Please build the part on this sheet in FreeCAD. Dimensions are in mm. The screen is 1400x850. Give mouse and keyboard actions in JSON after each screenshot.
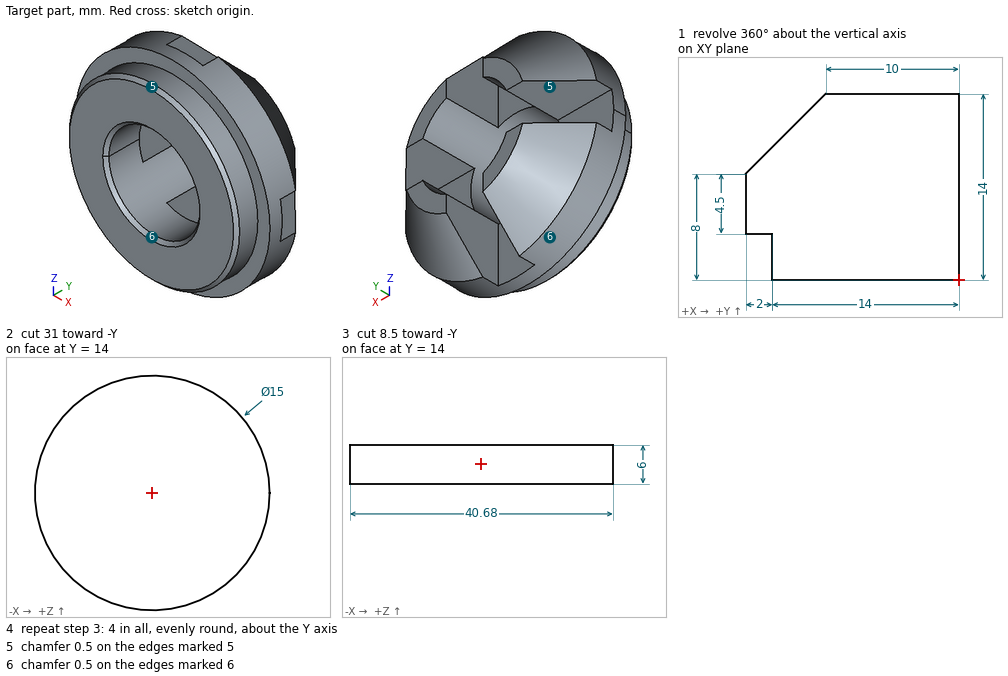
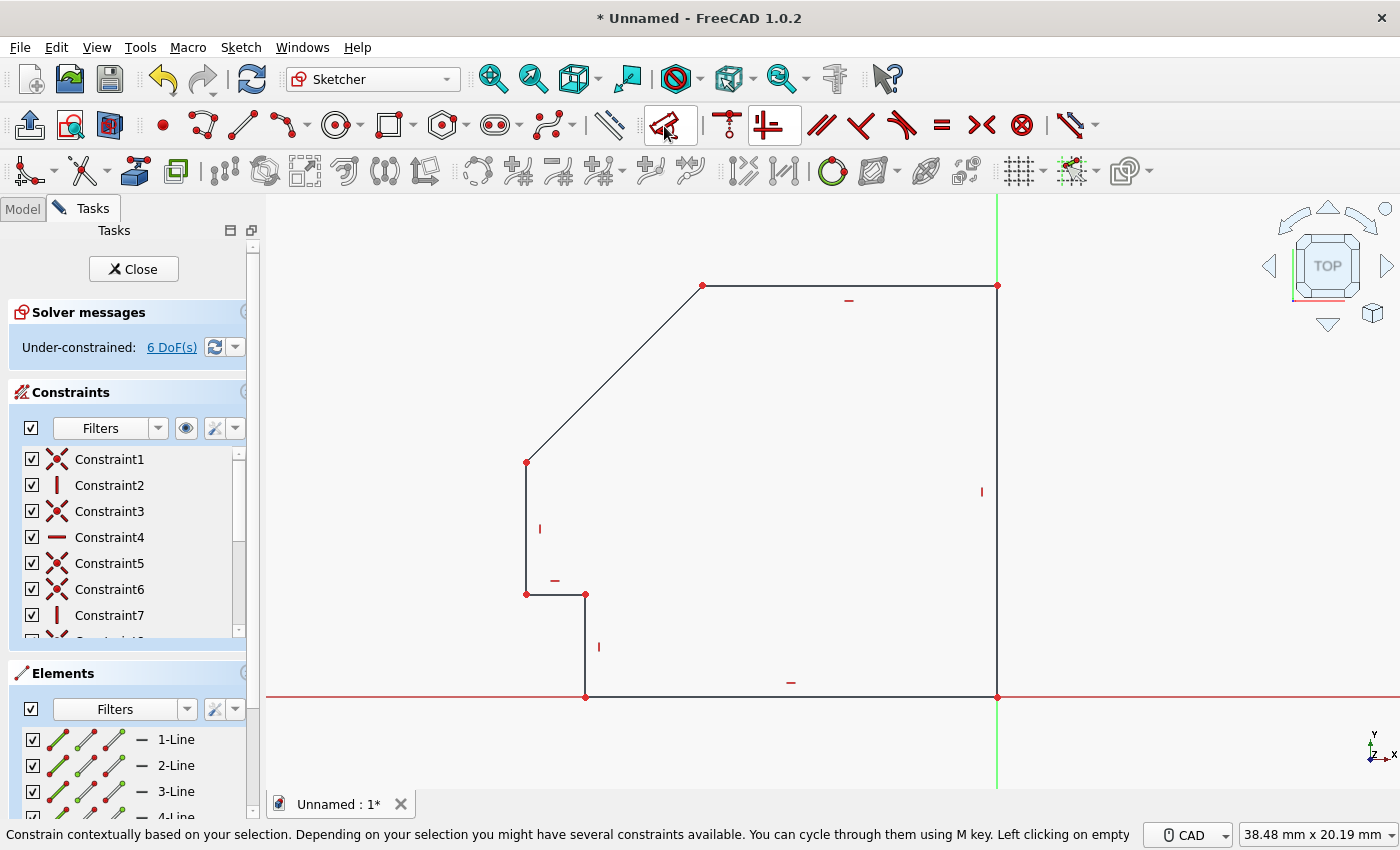
{"action": "left_click", "coordinate": [544, 595]}
{"action": "left_click", "coordinate": [555, 629]}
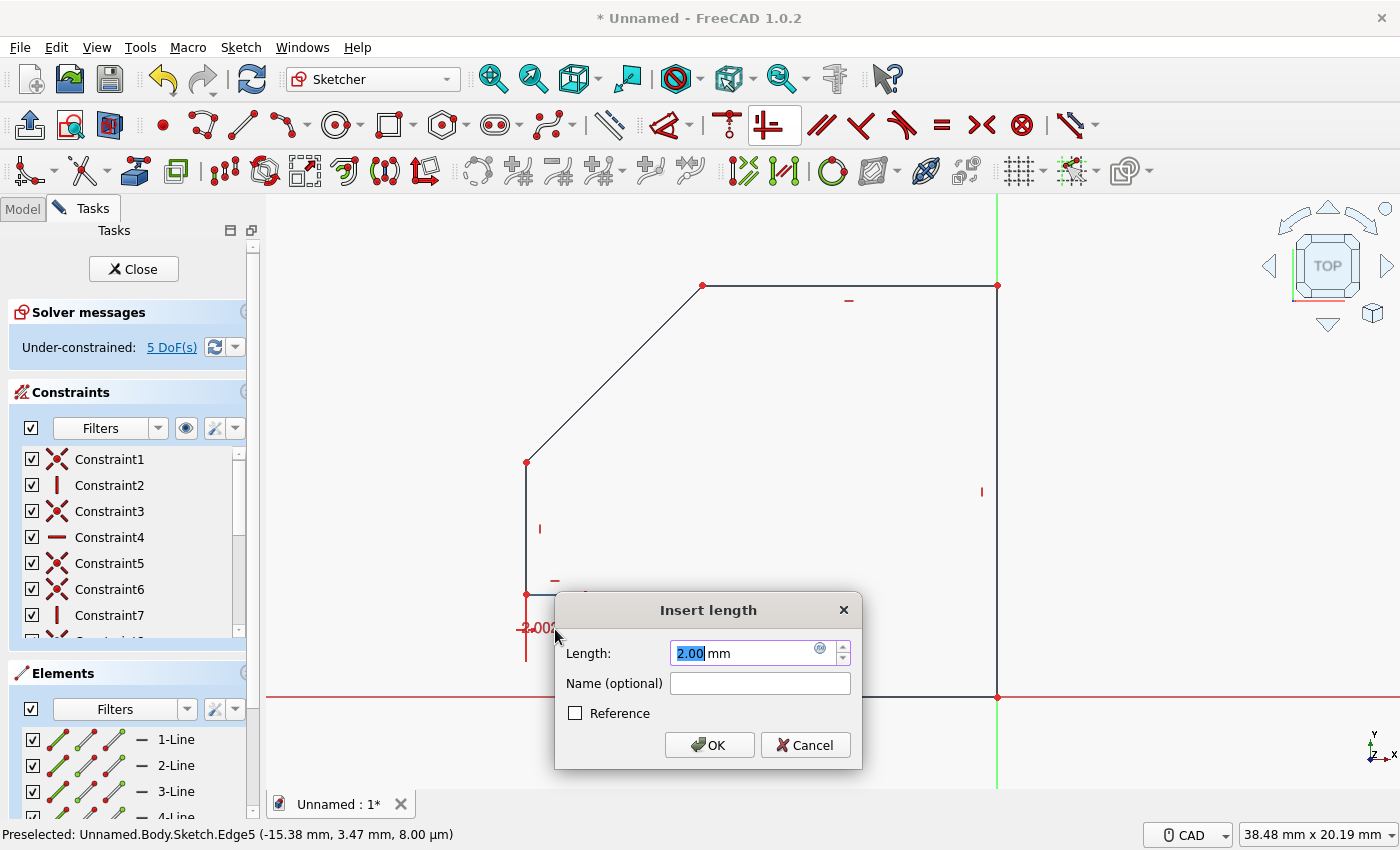
{"action": "type", "text": "2"}
{"action": "key", "text": "Return"}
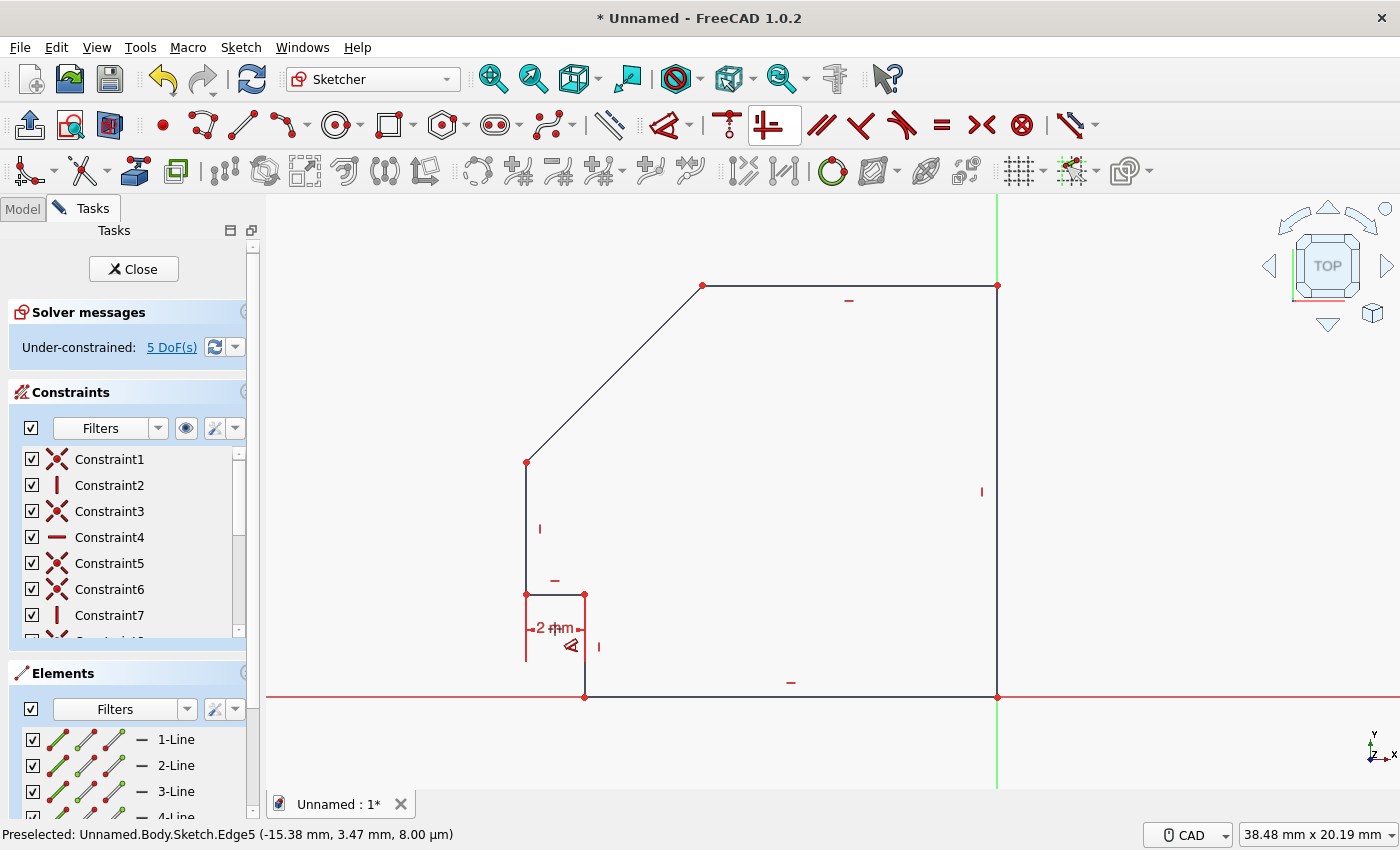
{"action": "left_click", "coordinate": [997, 574]}
{"action": "left_click", "coordinate": [1031, 492]}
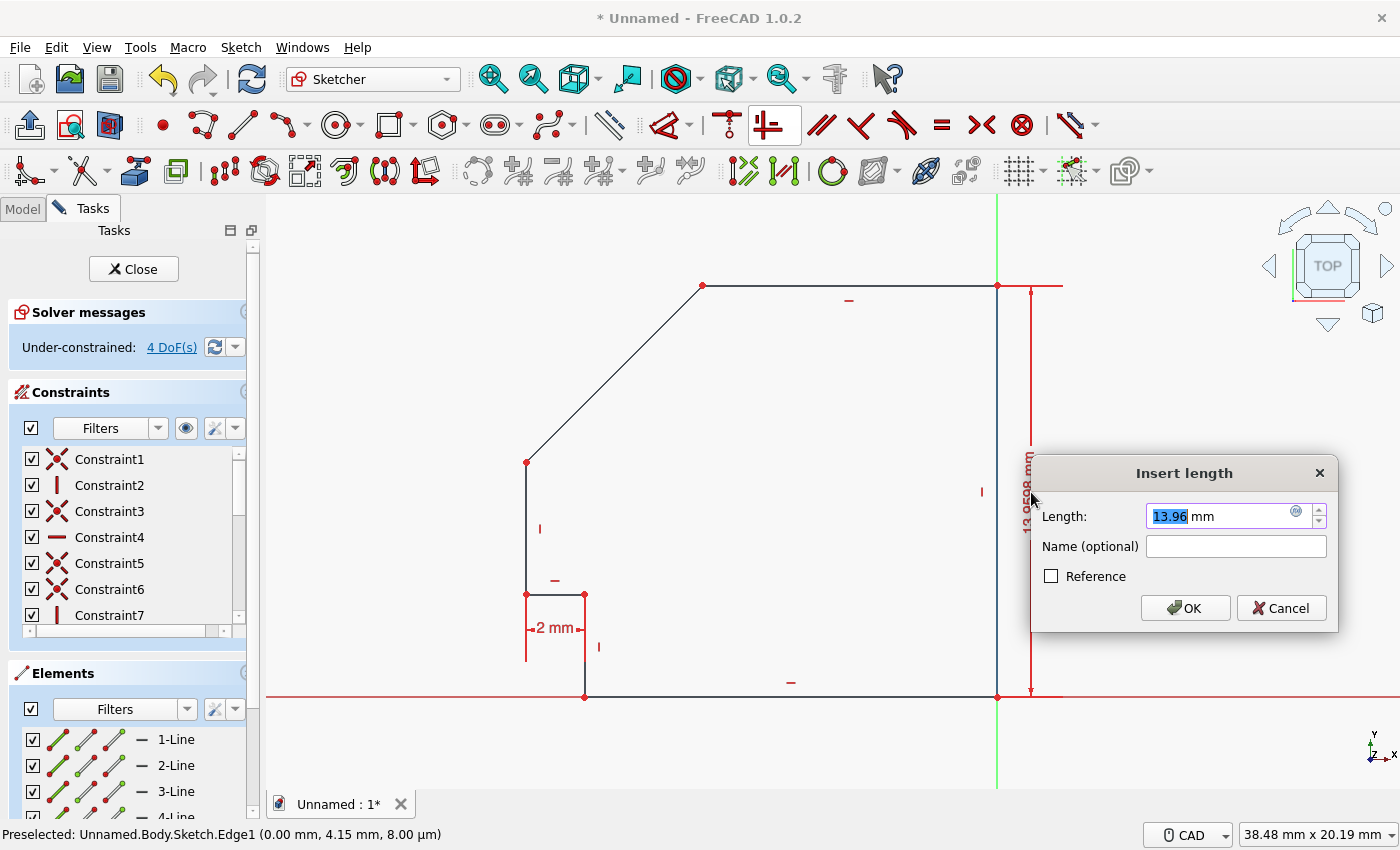
{"action": "type", "text": "14"}
{"action": "key", "text": "Return"}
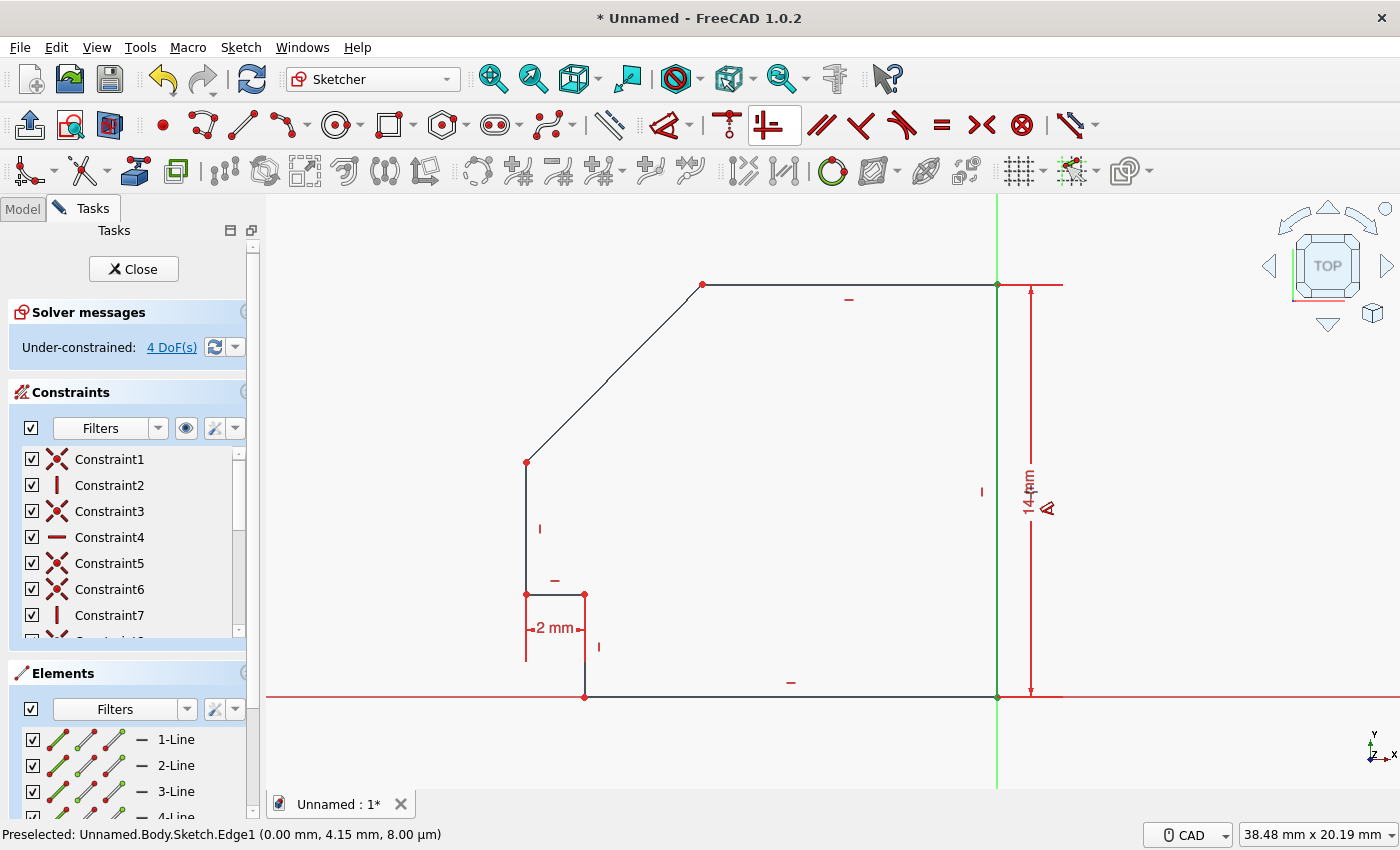
{"action": "left_click", "coordinate": [909, 285]}
{"action": "left_click", "coordinate": [850, 251]}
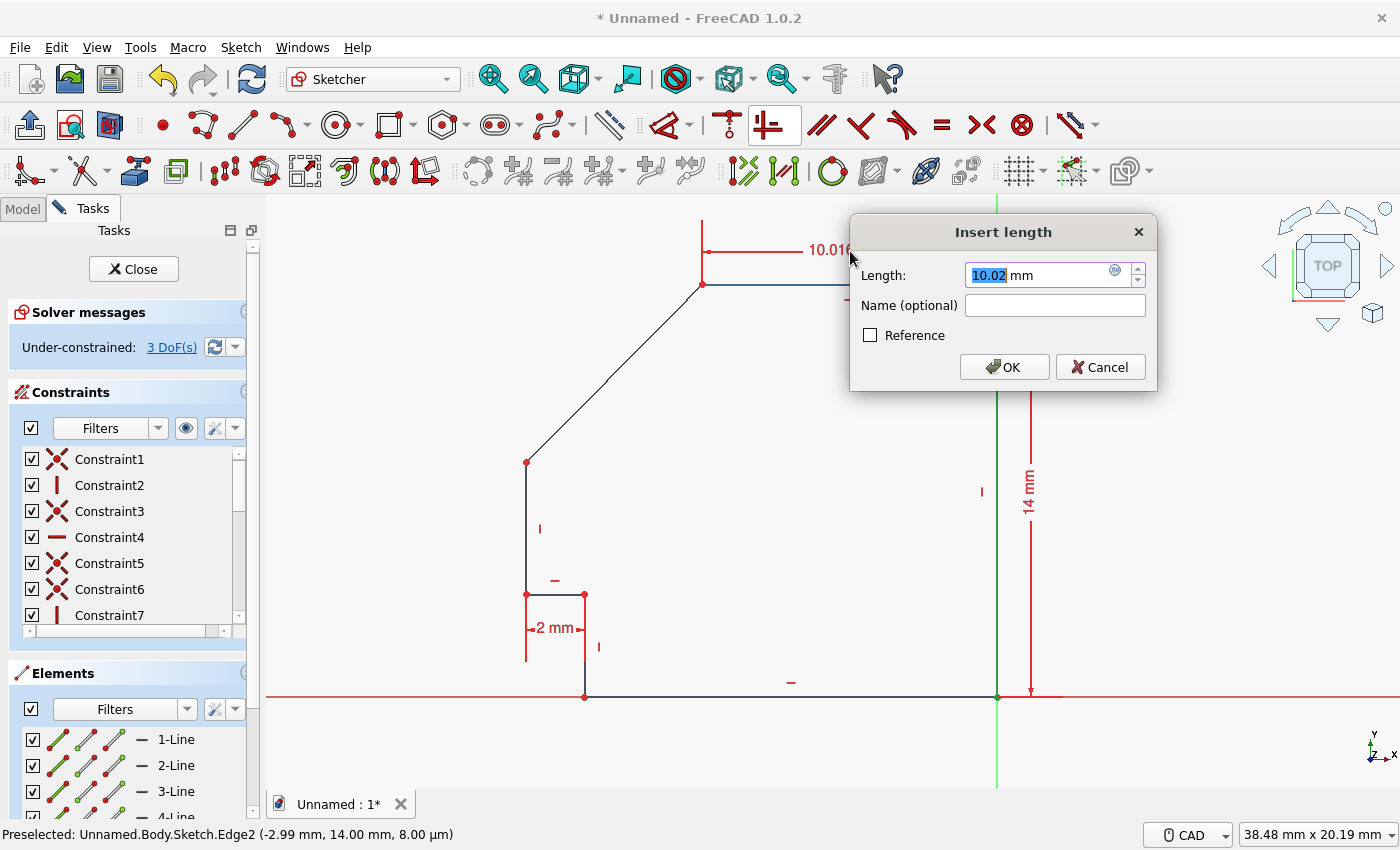
{"action": "type", "text": "10"}
{"action": "key", "text": "Return"}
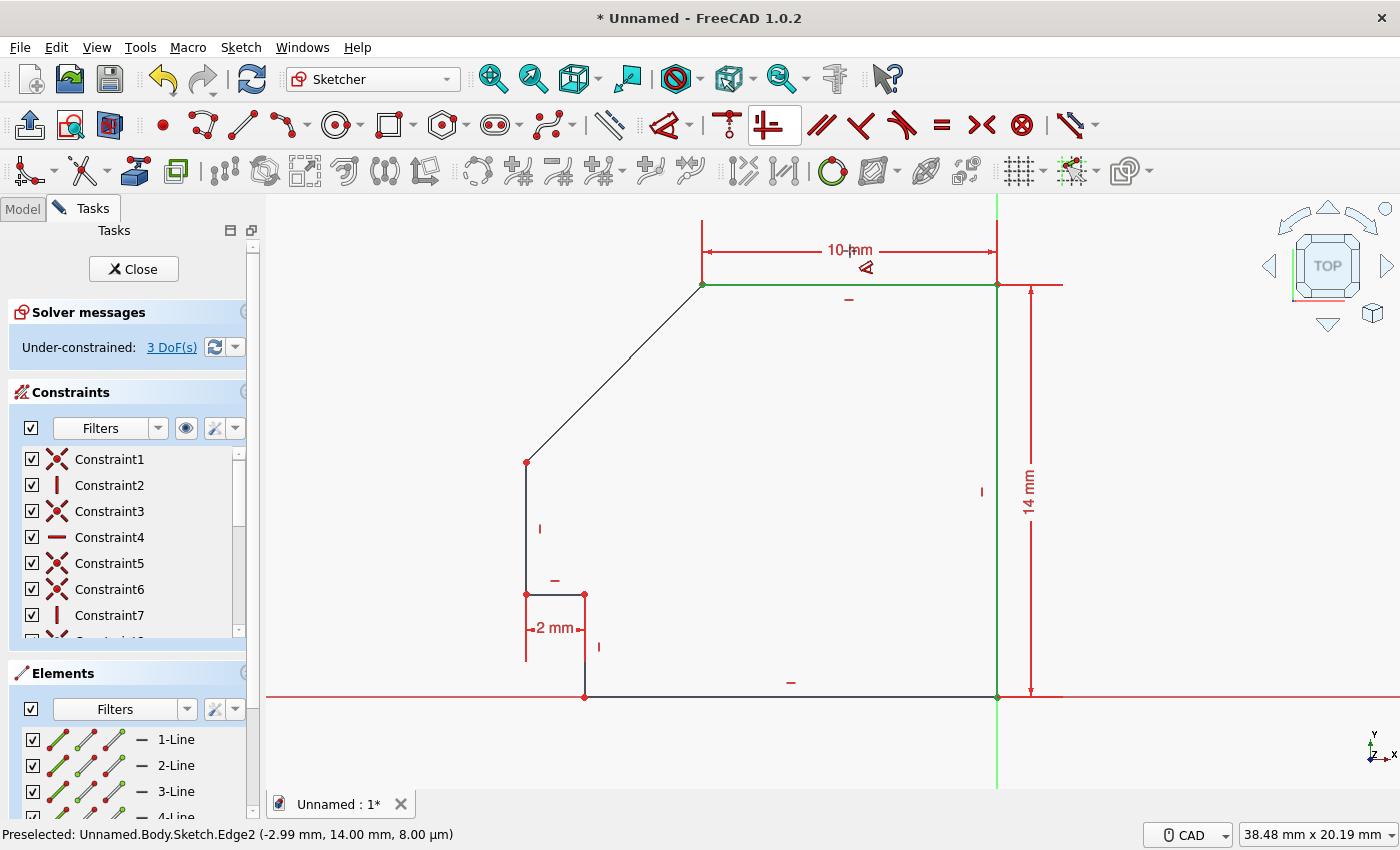
{"action": "left_click", "coordinate": [709, 697]}
{"action": "left_click", "coordinate": [791, 731]}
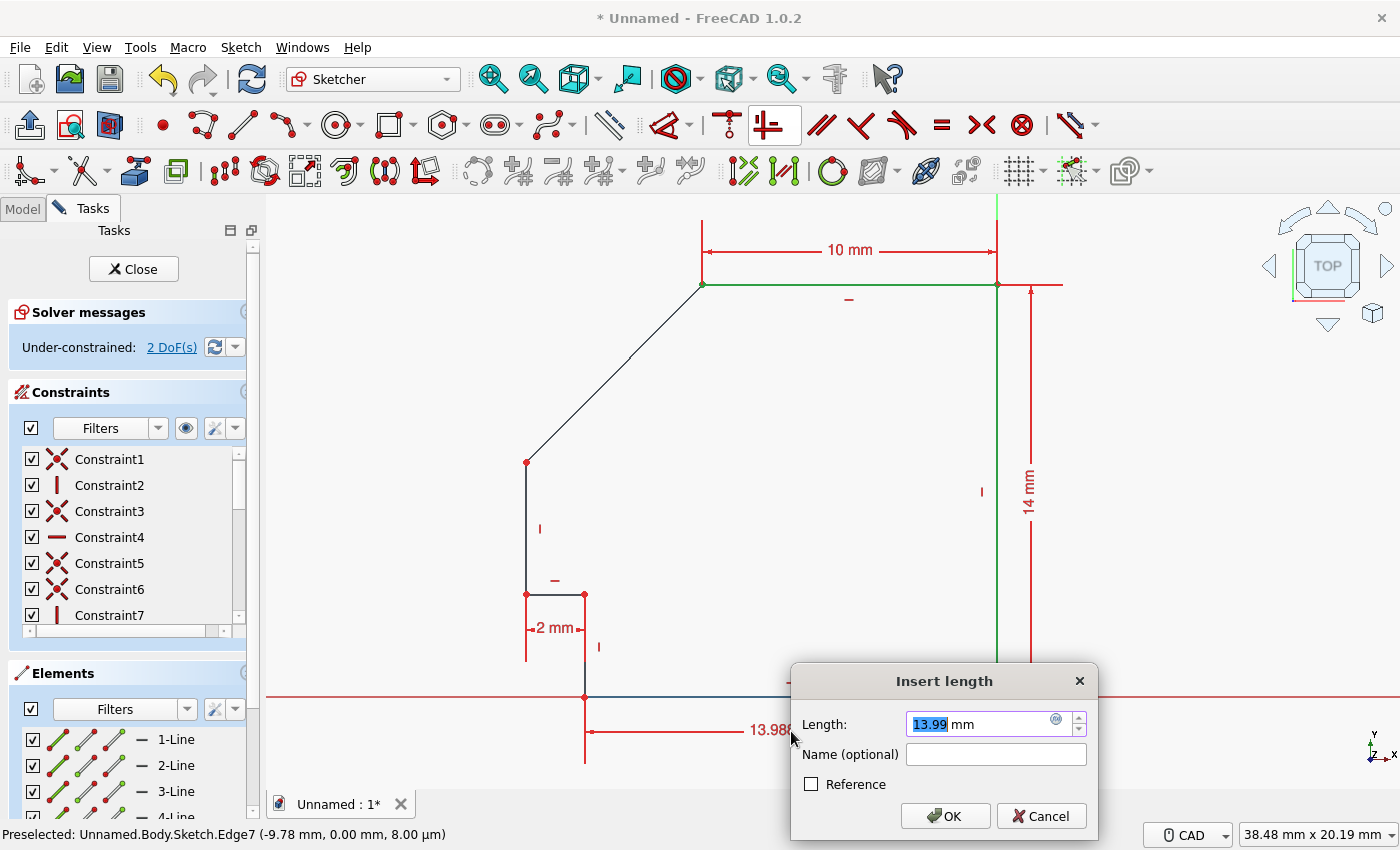
{"action": "type", "text": "14"}
{"action": "key", "text": "Return"}